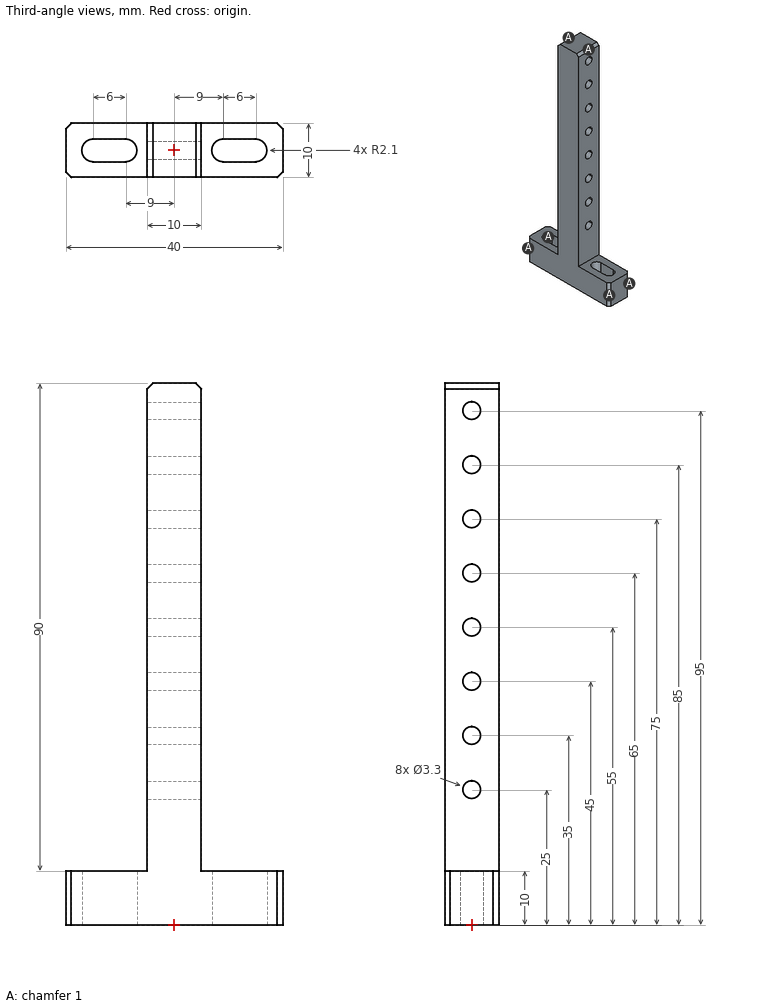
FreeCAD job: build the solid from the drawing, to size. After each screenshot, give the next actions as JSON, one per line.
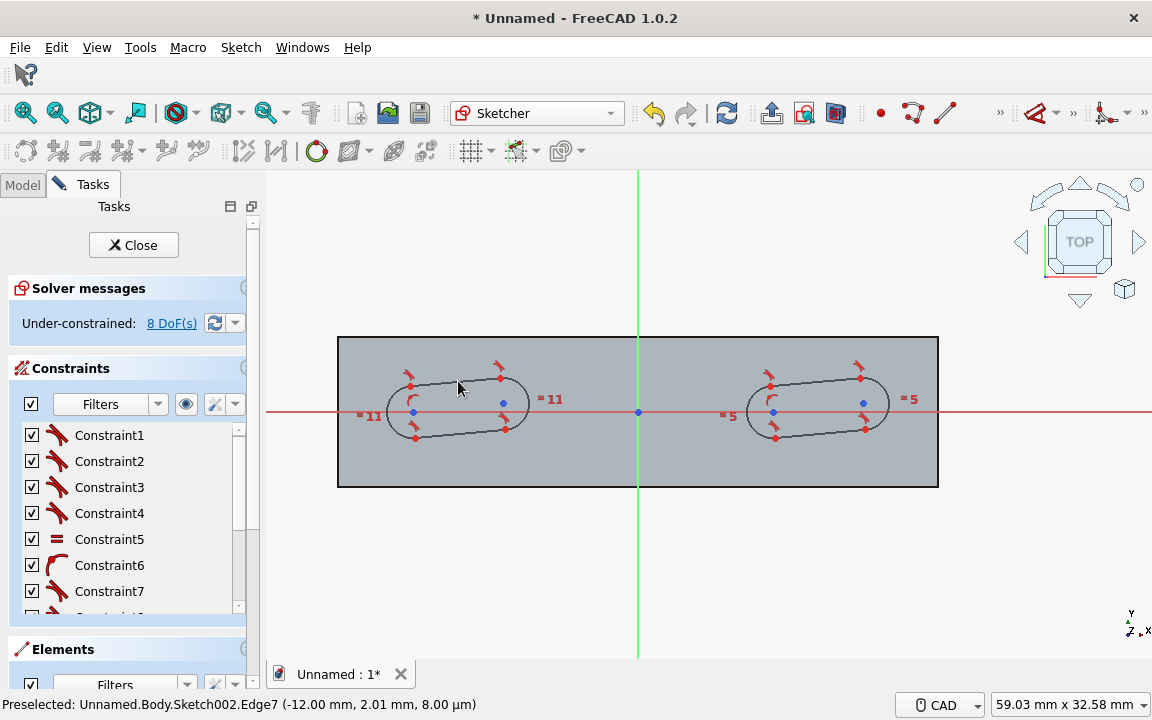
{"action": "left_click", "coordinate": [798, 384]}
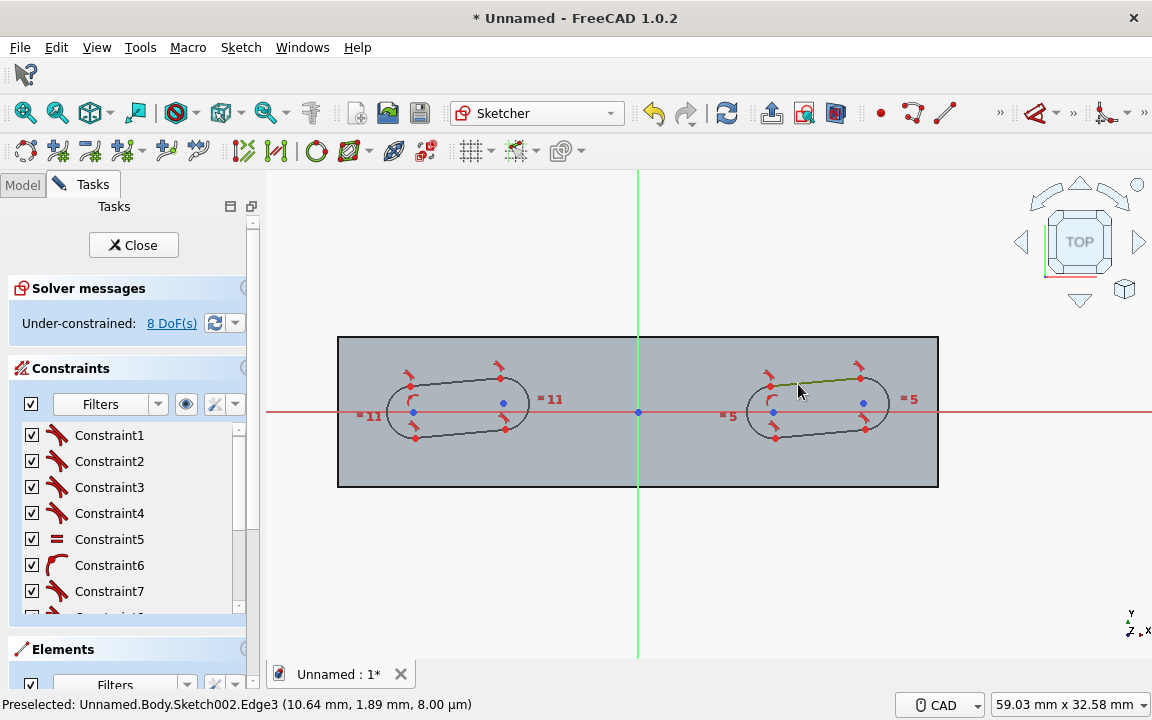
{"action": "key", "text": "h"}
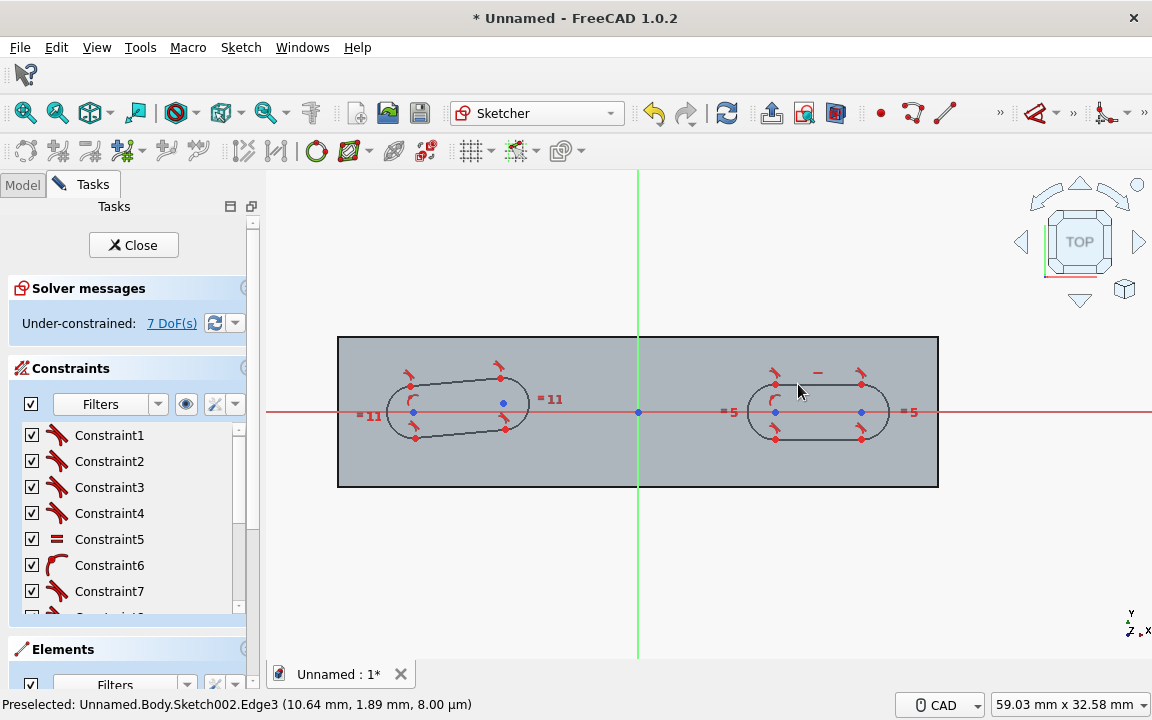
{"action": "left_click", "coordinate": [438, 384]}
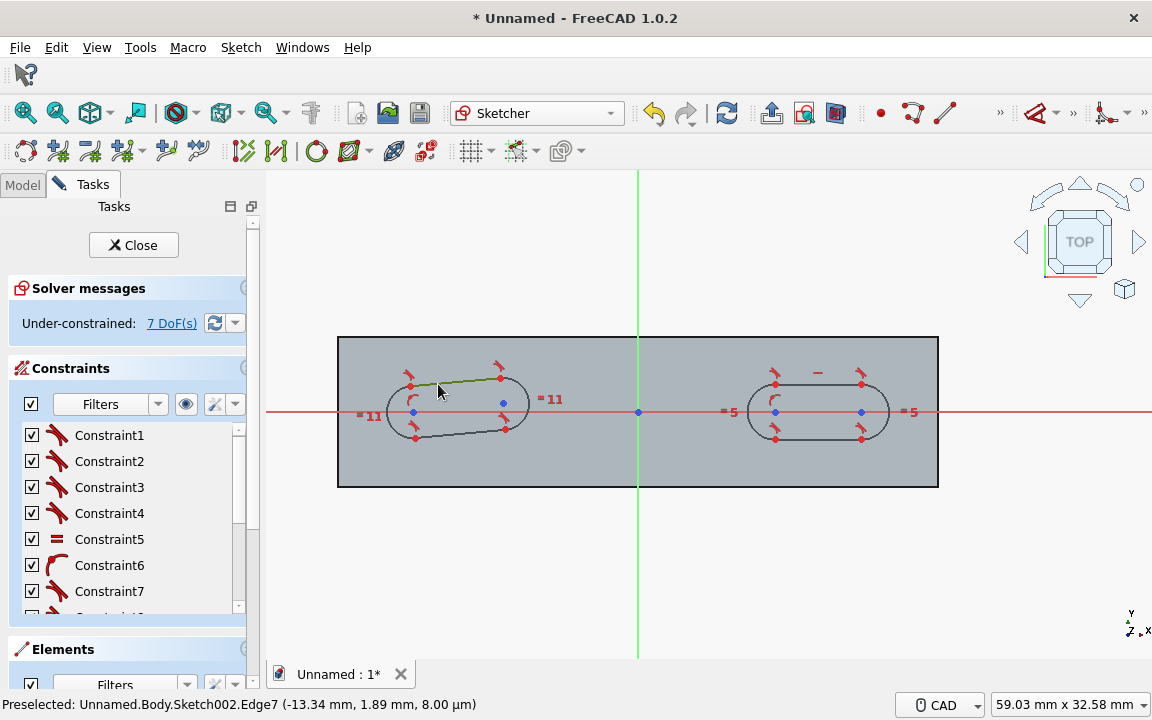
{"action": "key", "text": "h"}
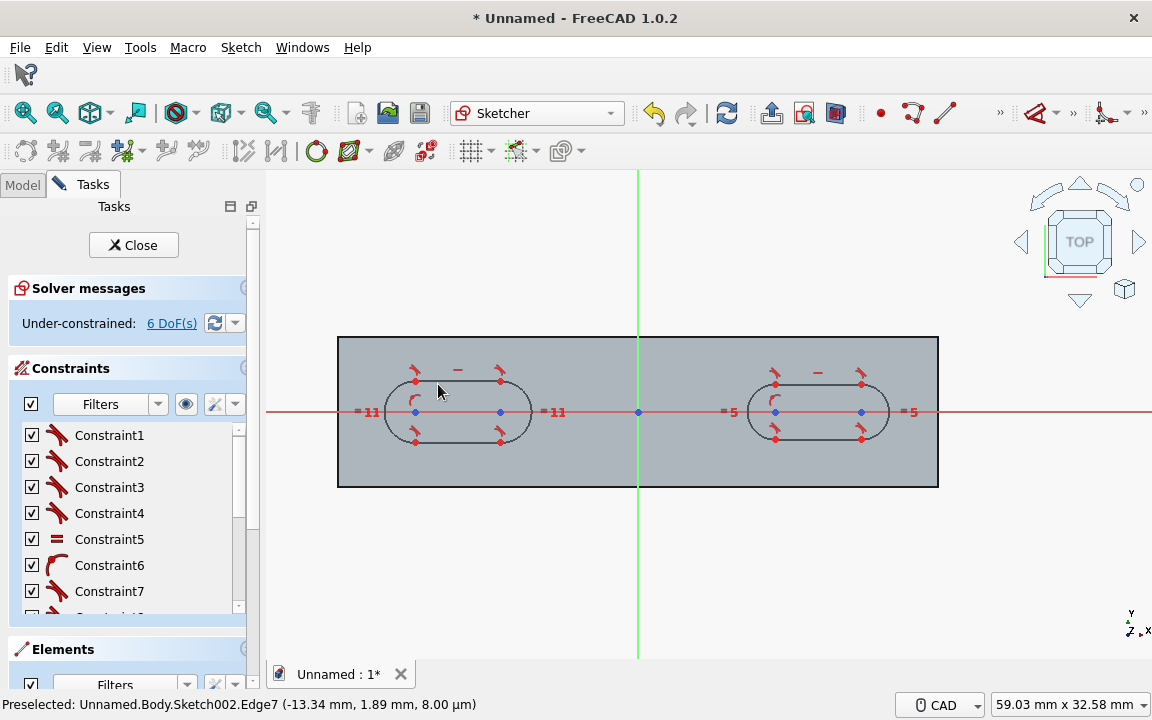
{"action": "left_click", "coordinate": [753, 396]}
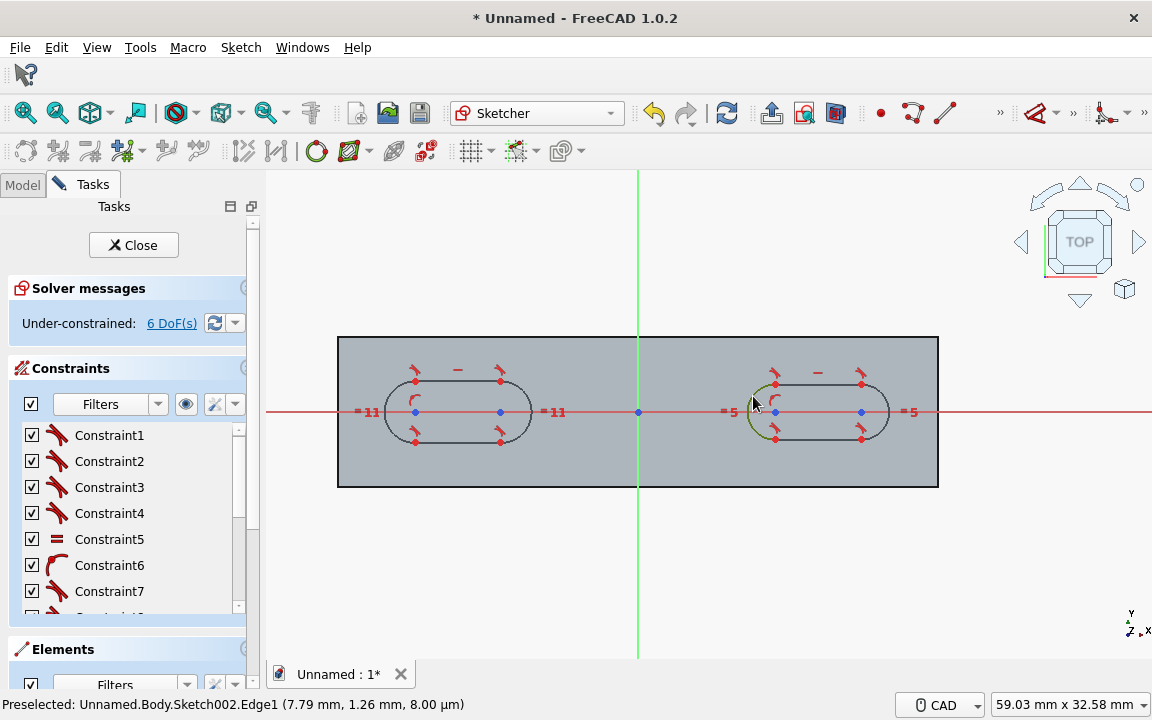
{"action": "left_click", "coordinate": [390, 394]}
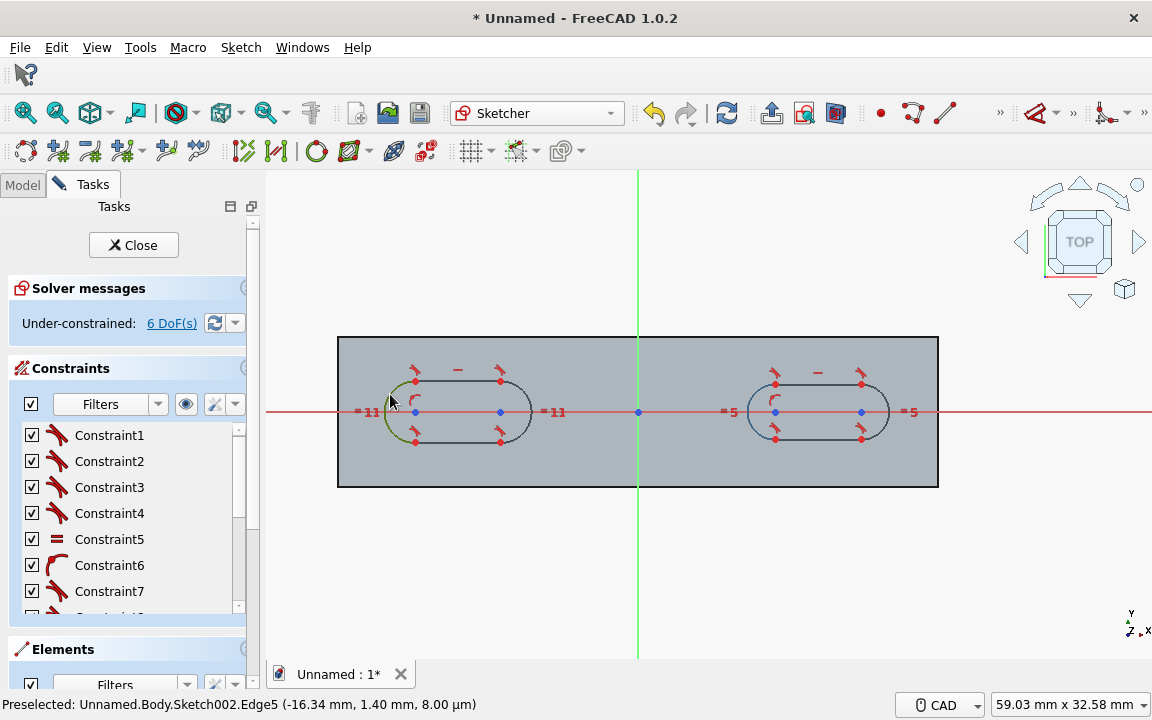
{"action": "key", "text": "e"}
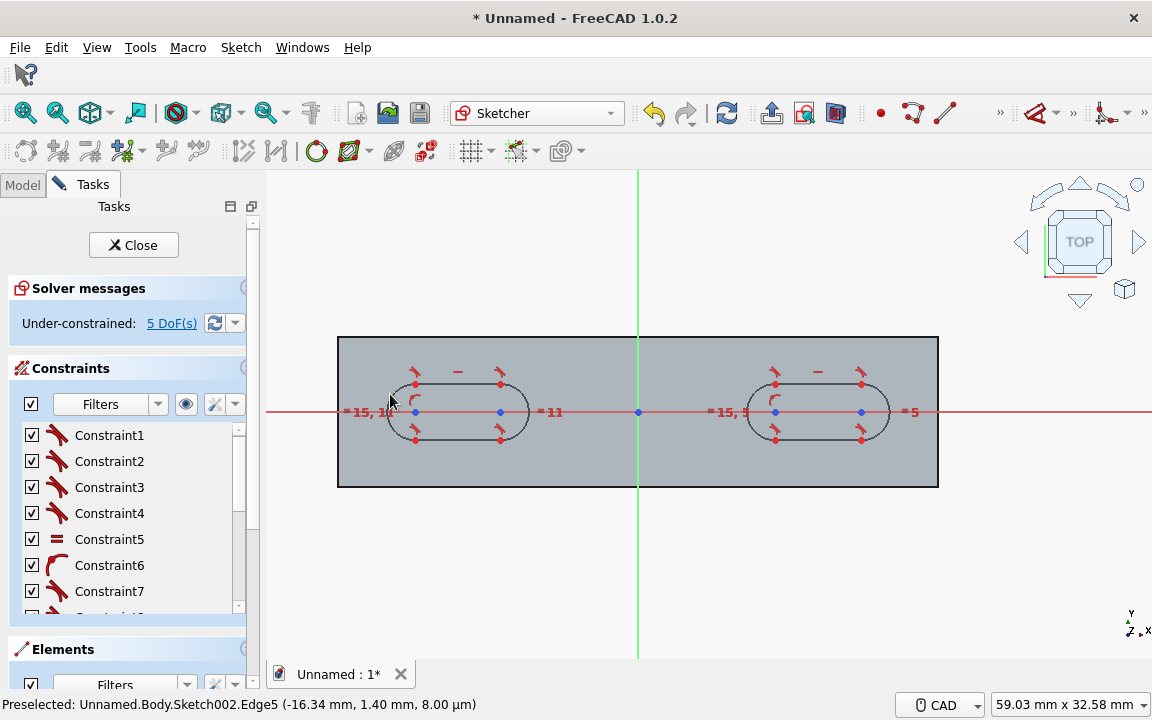
{"action": "left_click", "coordinate": [1036, 114]}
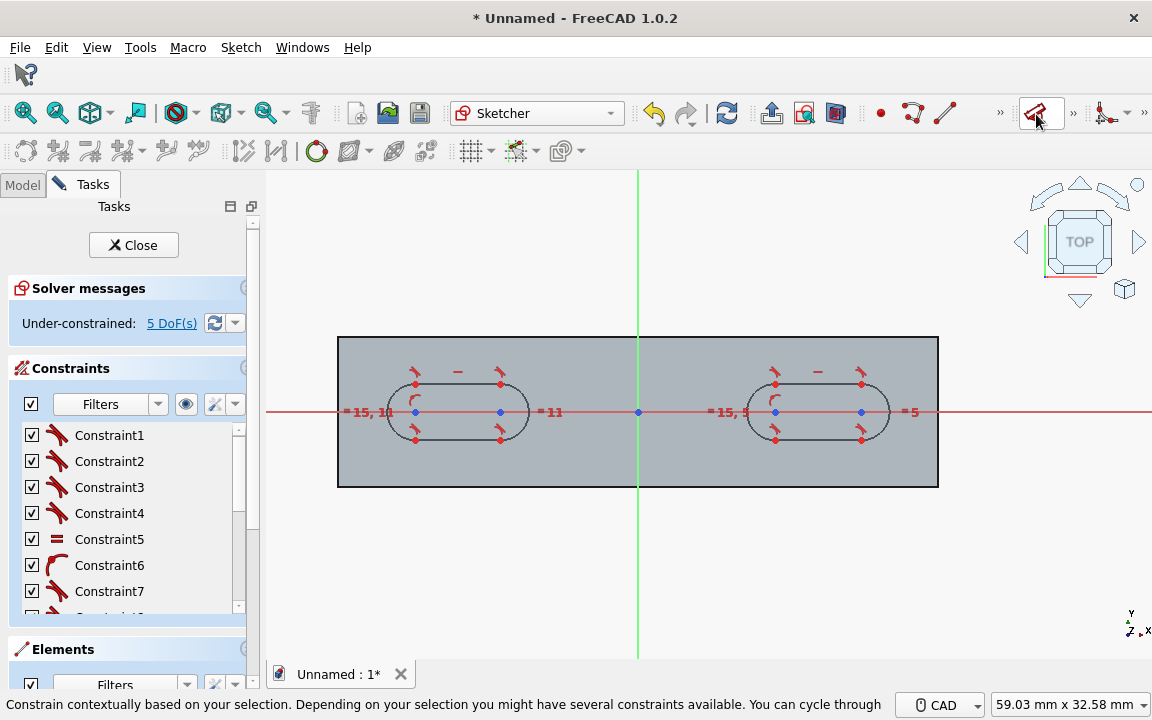
{"action": "scroll", "coordinate": [752, 396], "scroll_direction": "up", "scroll_amount": 2}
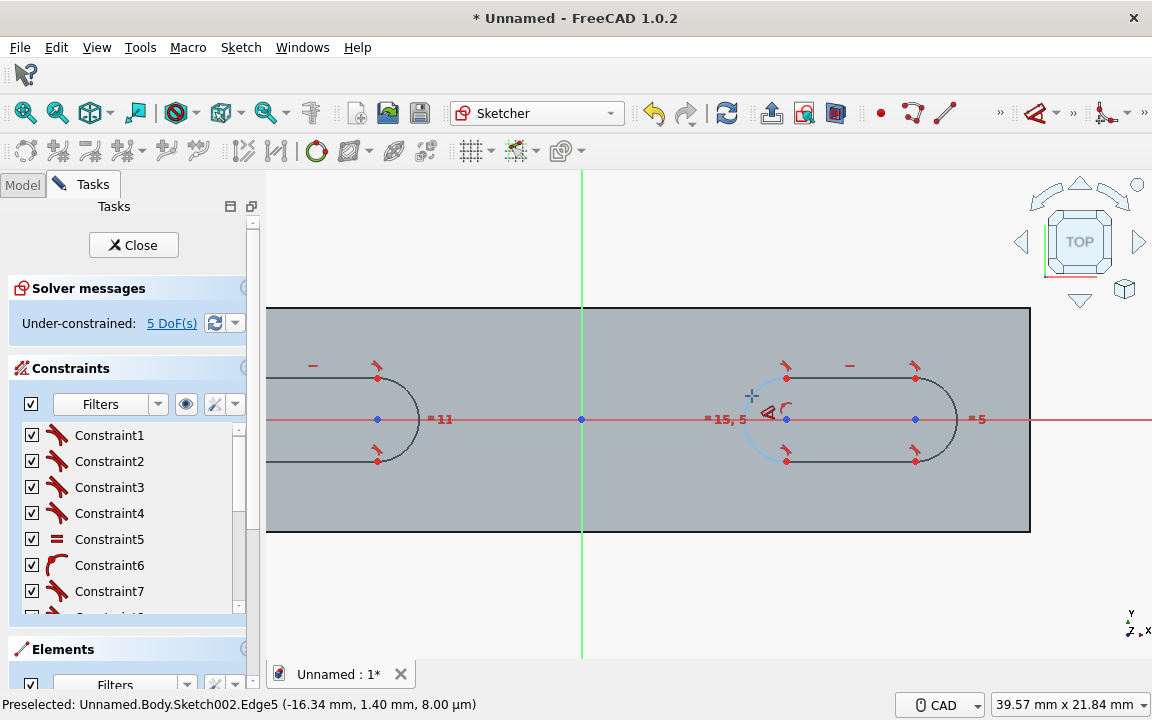
{"action": "left_click", "coordinate": [752, 395]}
{"action": "left_click", "coordinate": [726, 376]}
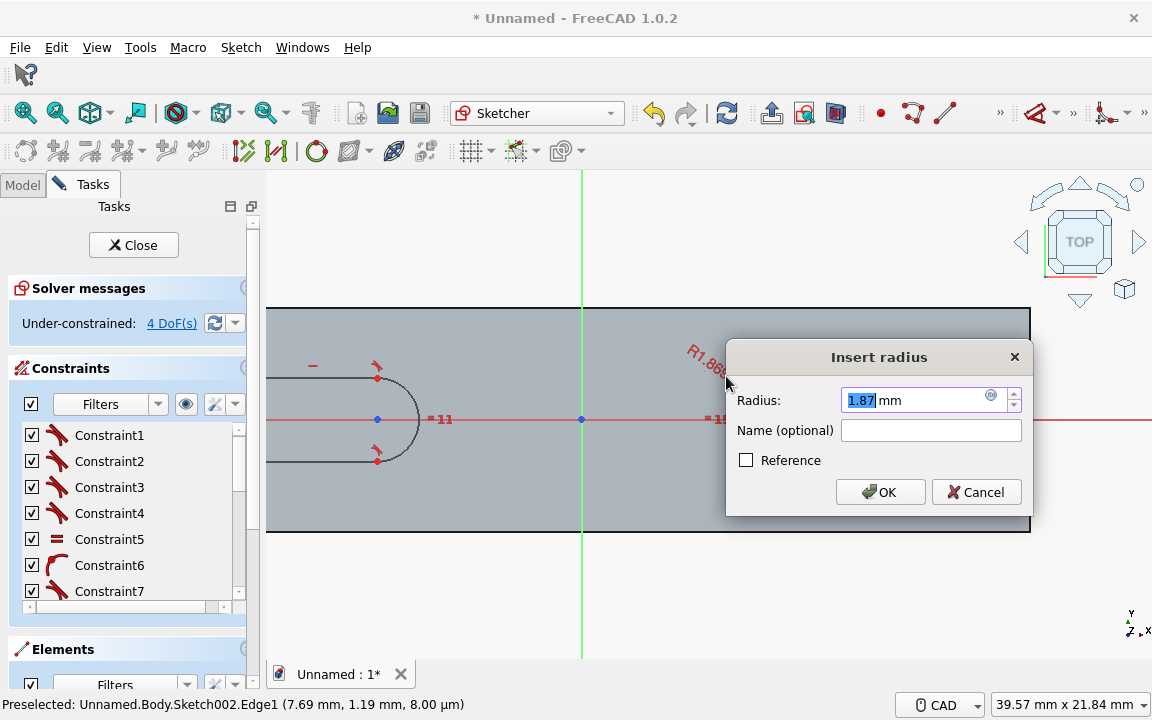
{"action": "type", "text": "2.1"}
{"action": "key", "text": "Return"}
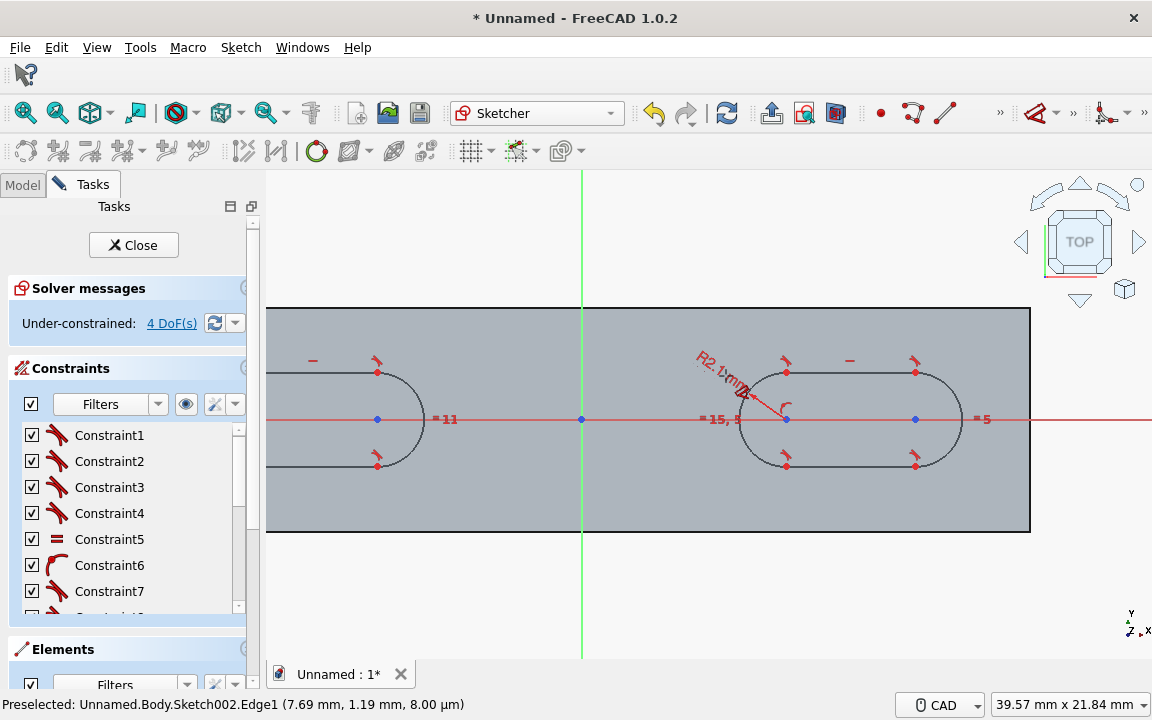
{"action": "left_click", "coordinate": [825, 373]}
{"action": "left_click", "coordinate": [851, 339]}